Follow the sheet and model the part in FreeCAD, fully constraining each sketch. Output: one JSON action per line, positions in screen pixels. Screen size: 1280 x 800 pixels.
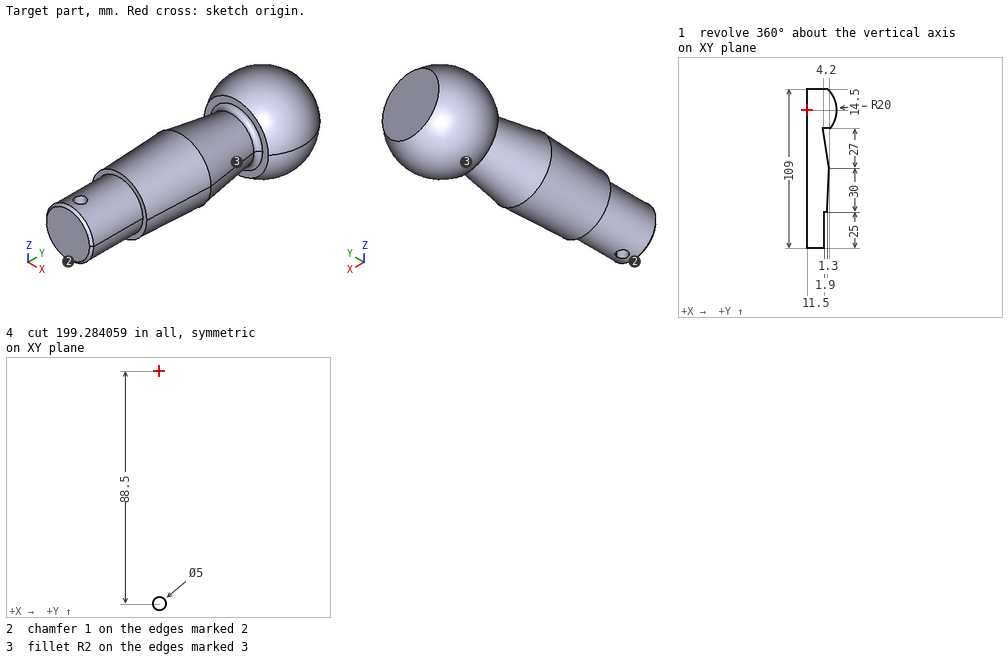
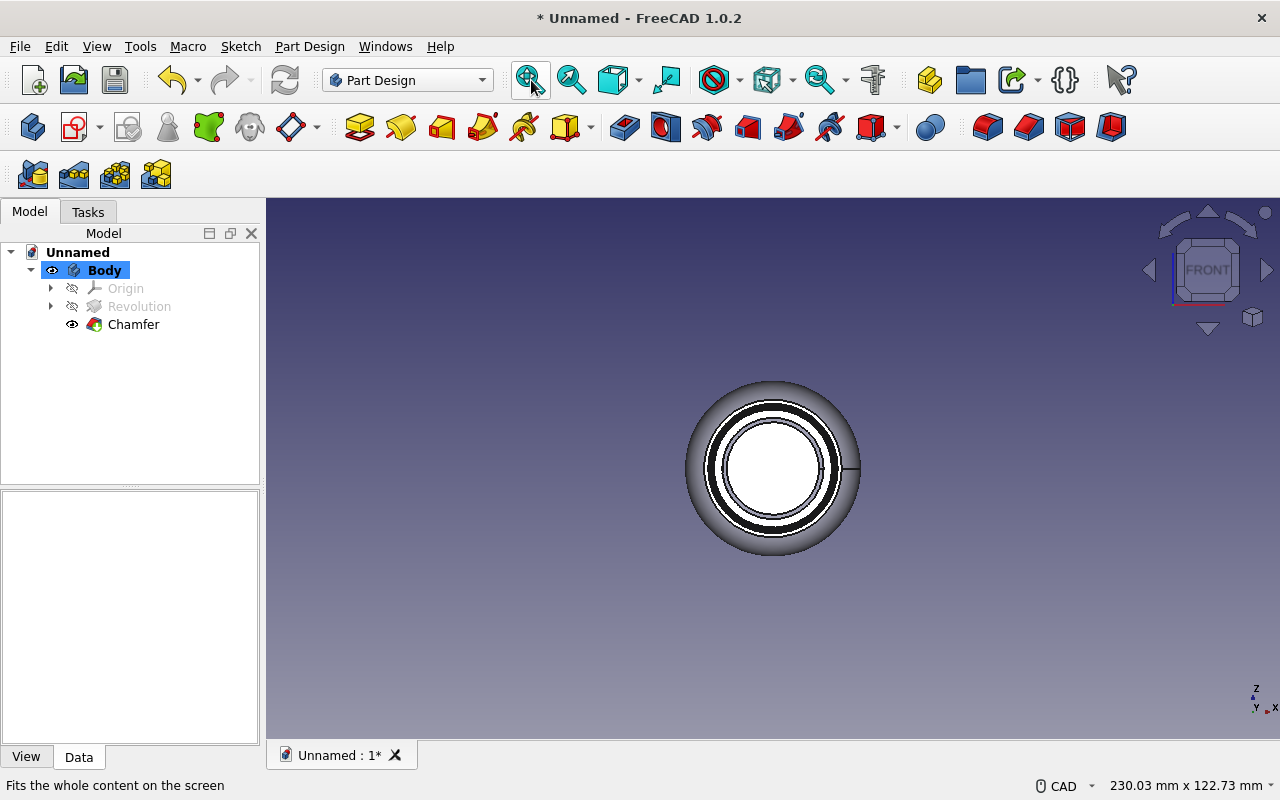
{"action": "key", "text": "3"}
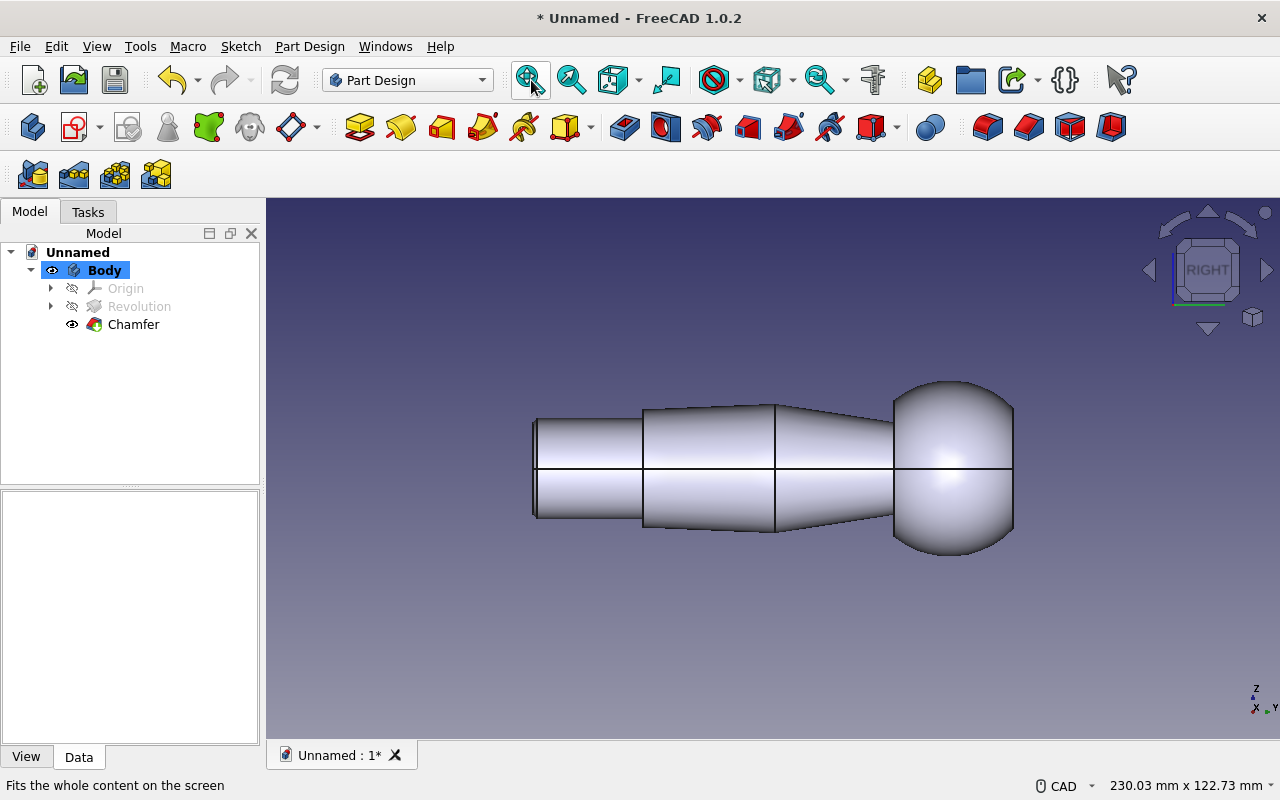
{"action": "key", "text": "5"}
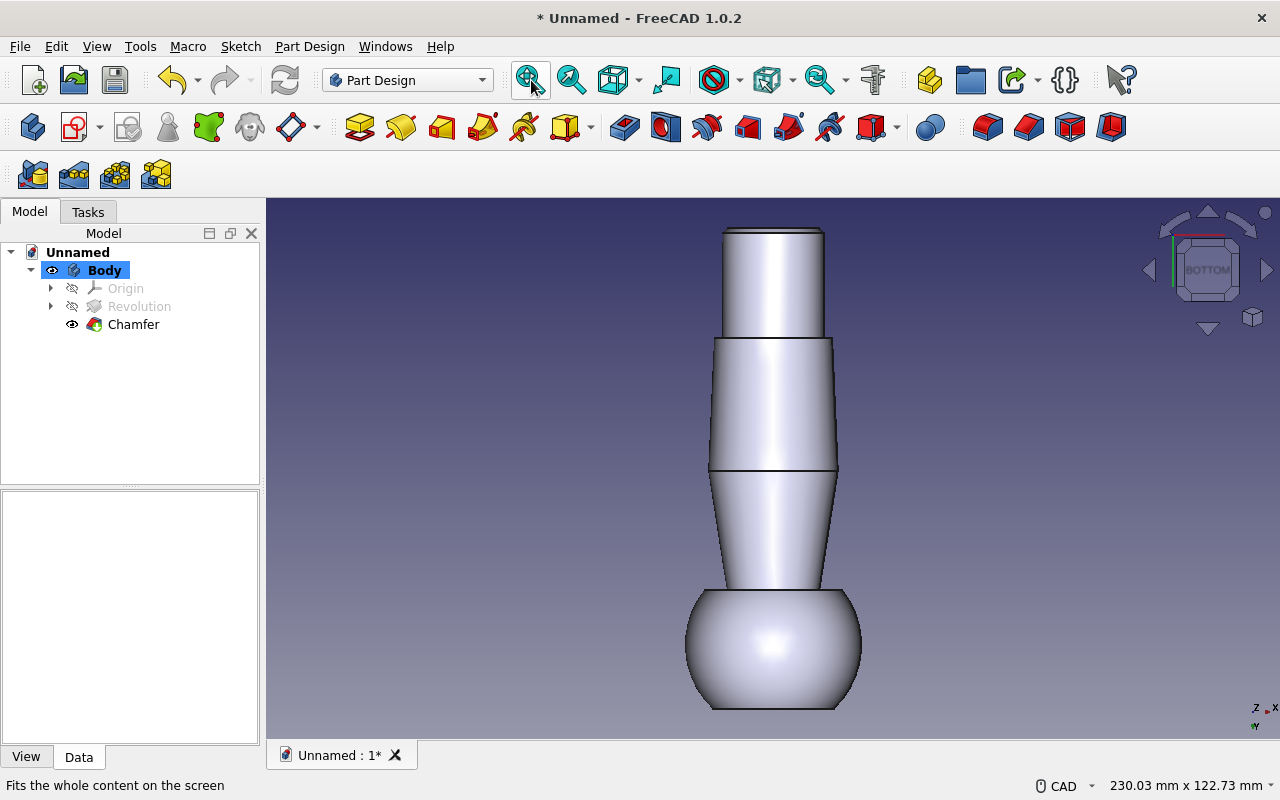
{"action": "key", "text": "4"}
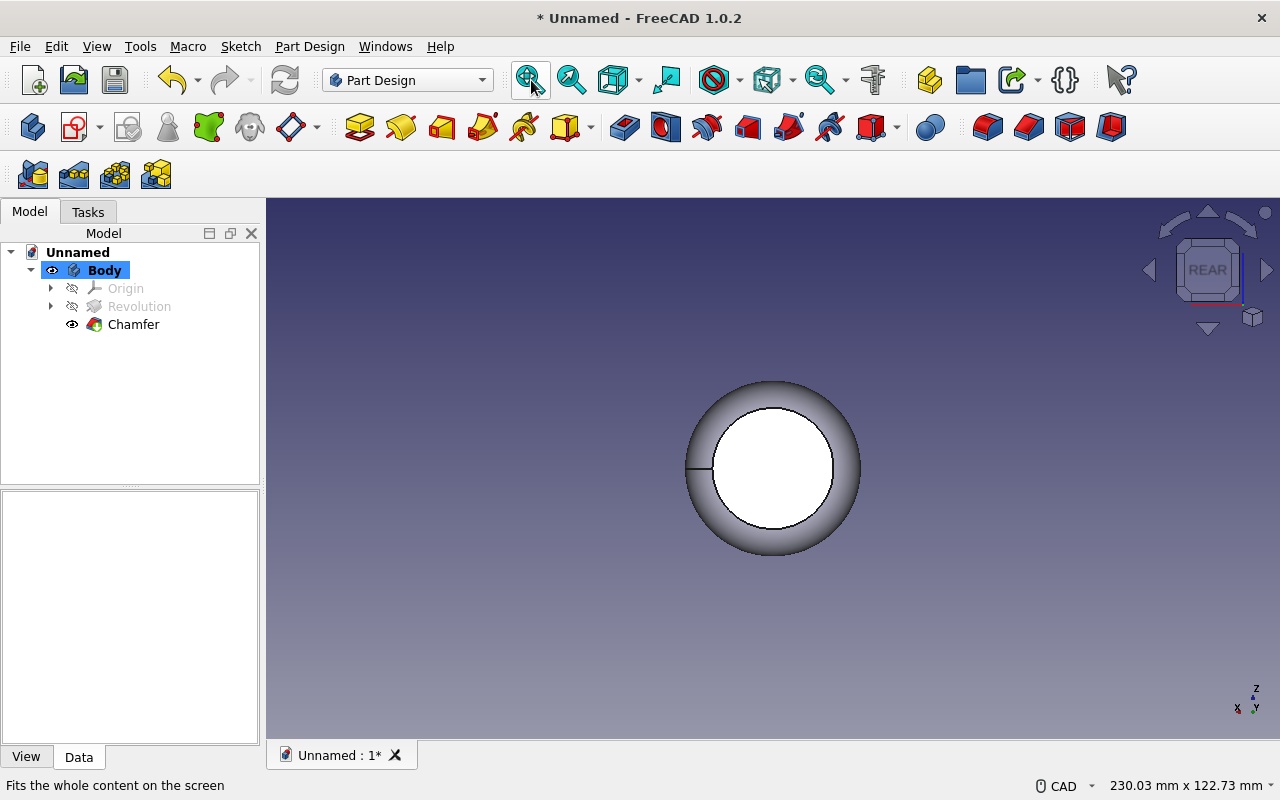
{"action": "left_click", "coordinate": [531, 80]}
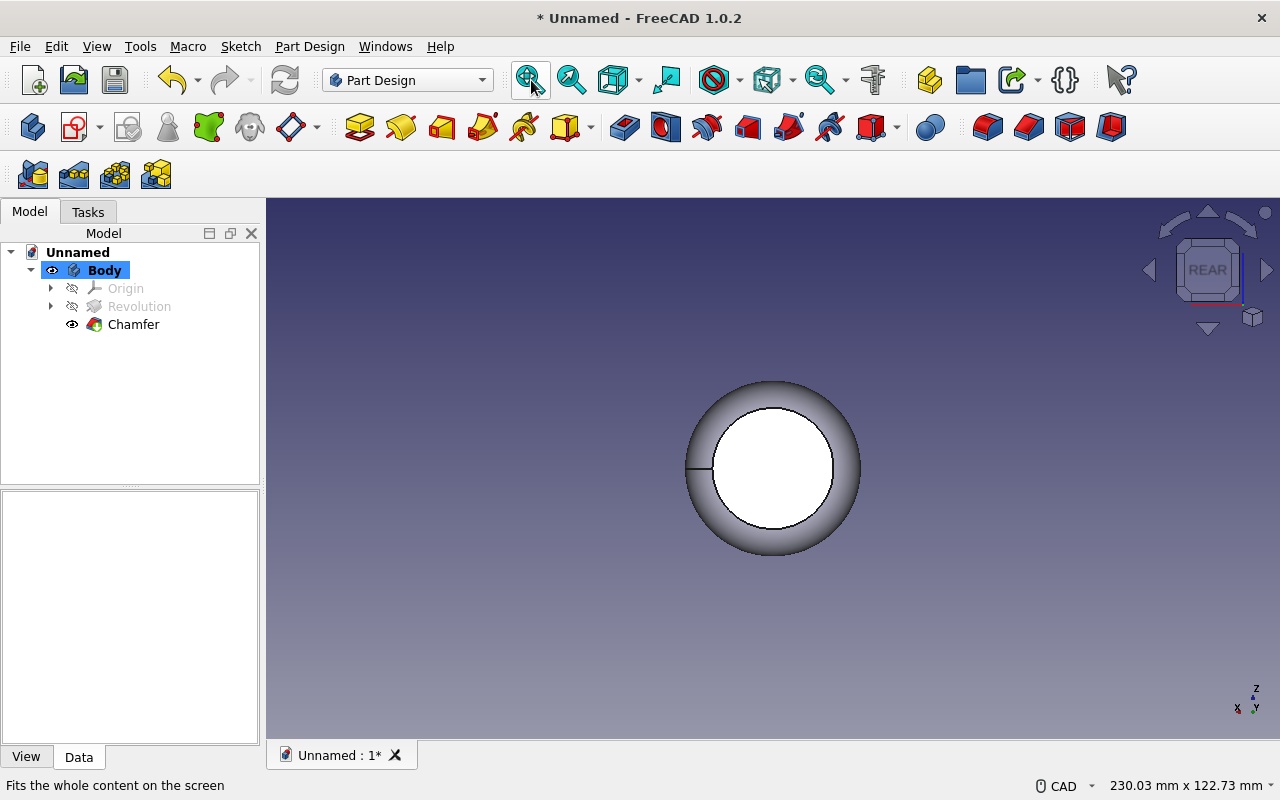
{"action": "key", "text": "6"}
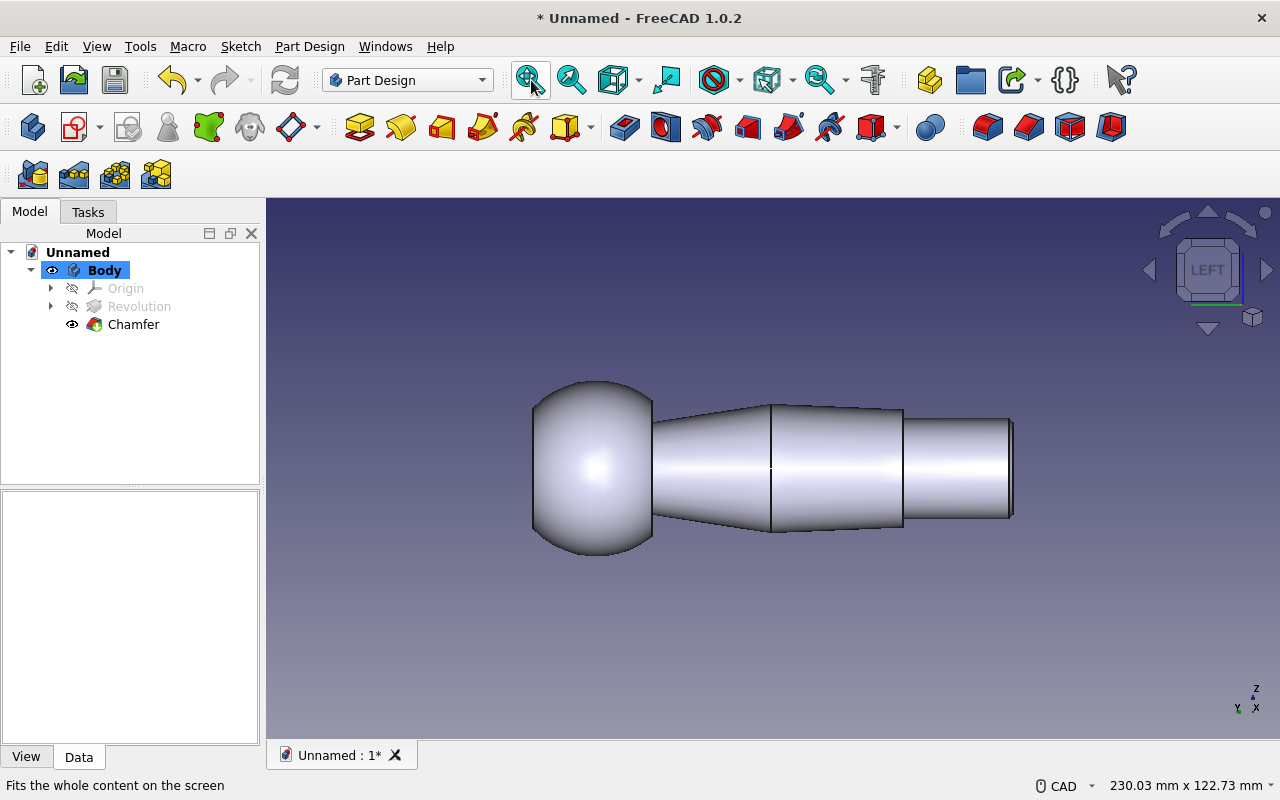
{"action": "key", "text": "v 3"}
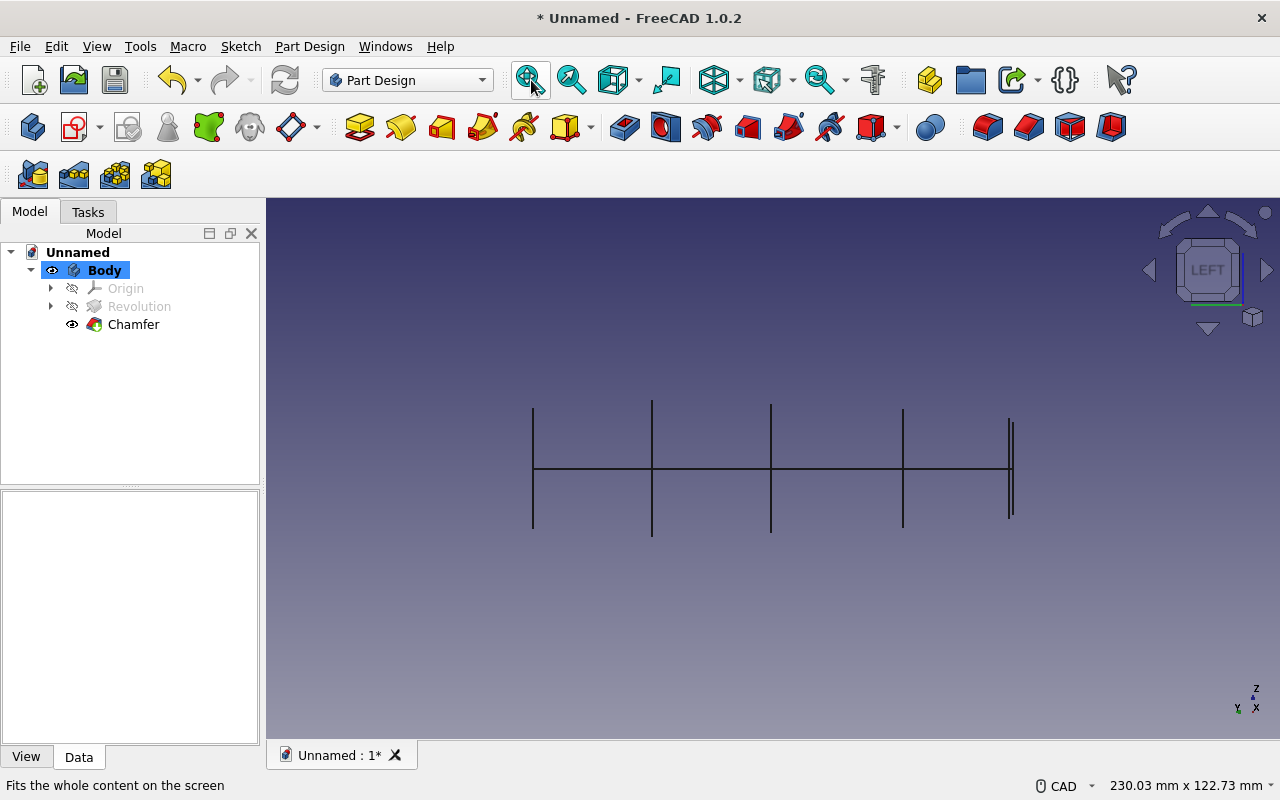
{"action": "key", "text": "0"}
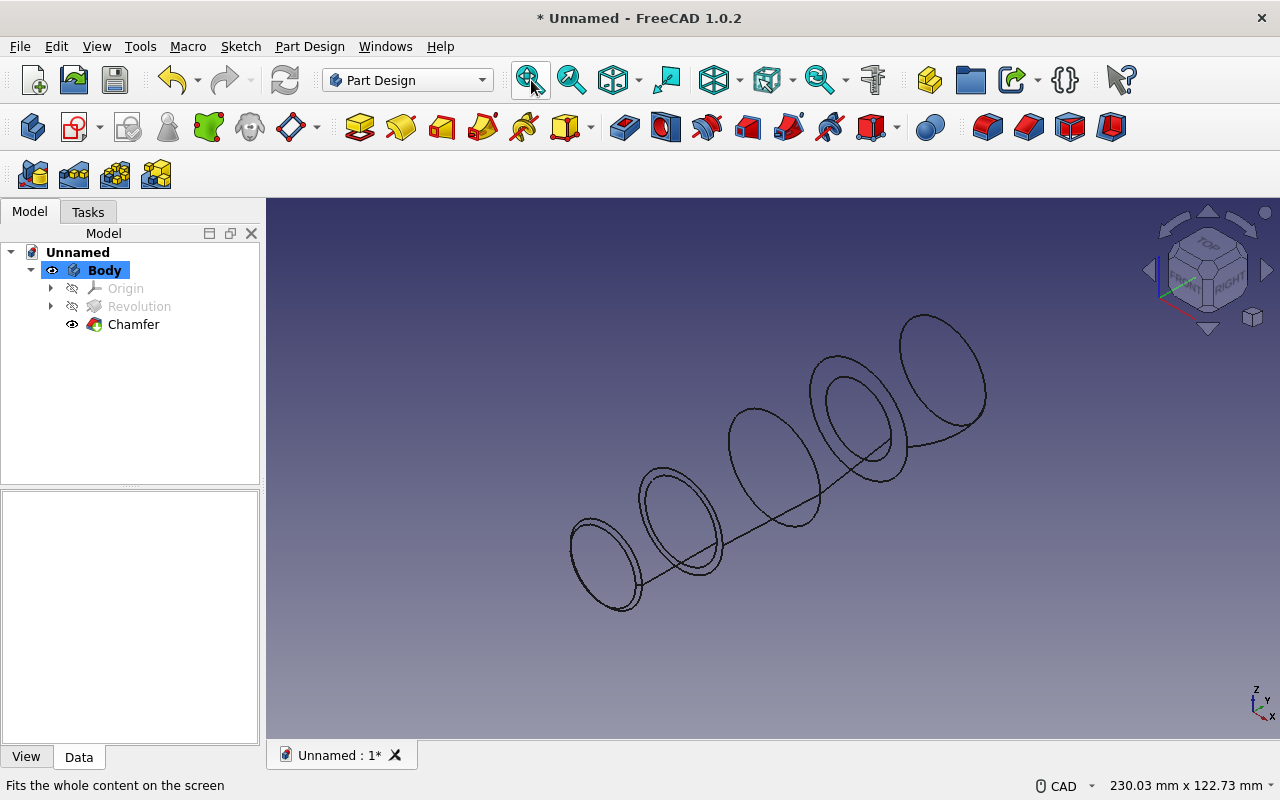
{"action": "left_click", "coordinate": [826, 399]}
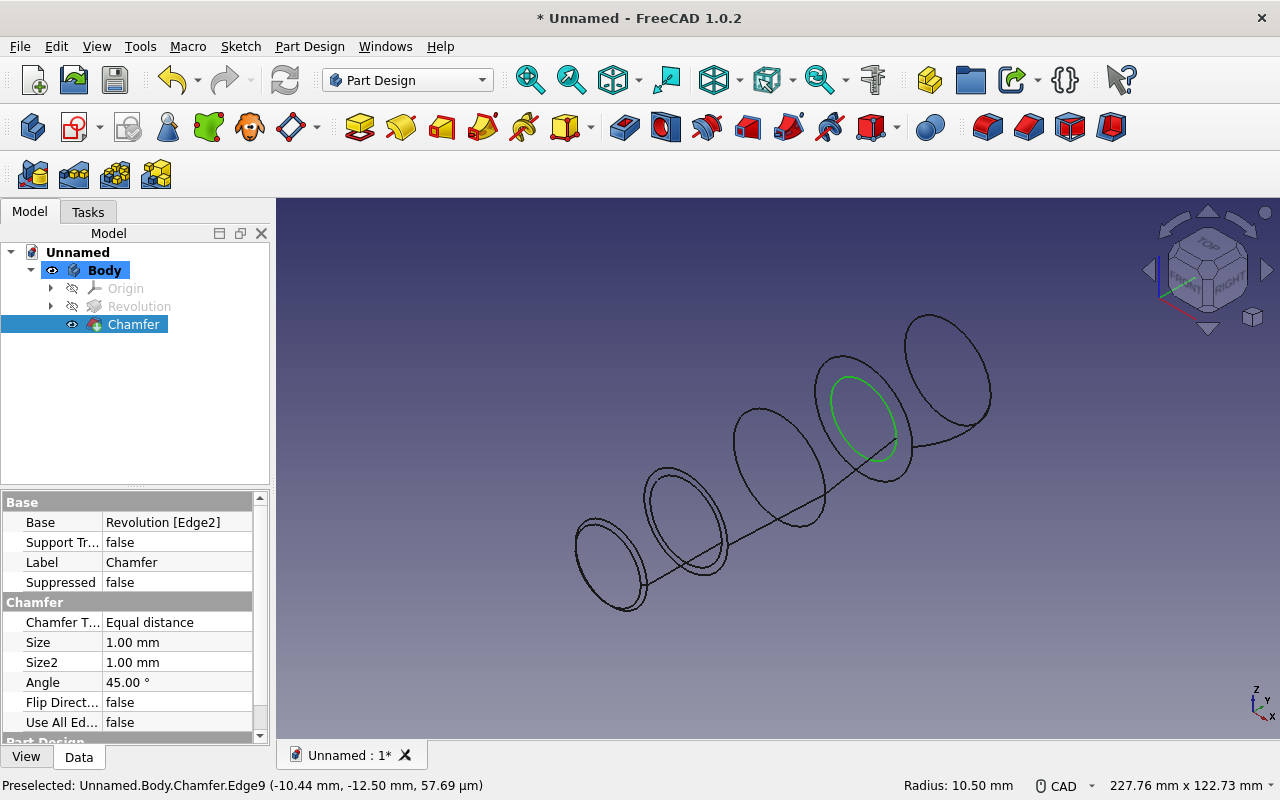
{"action": "key", "text": "v 1"}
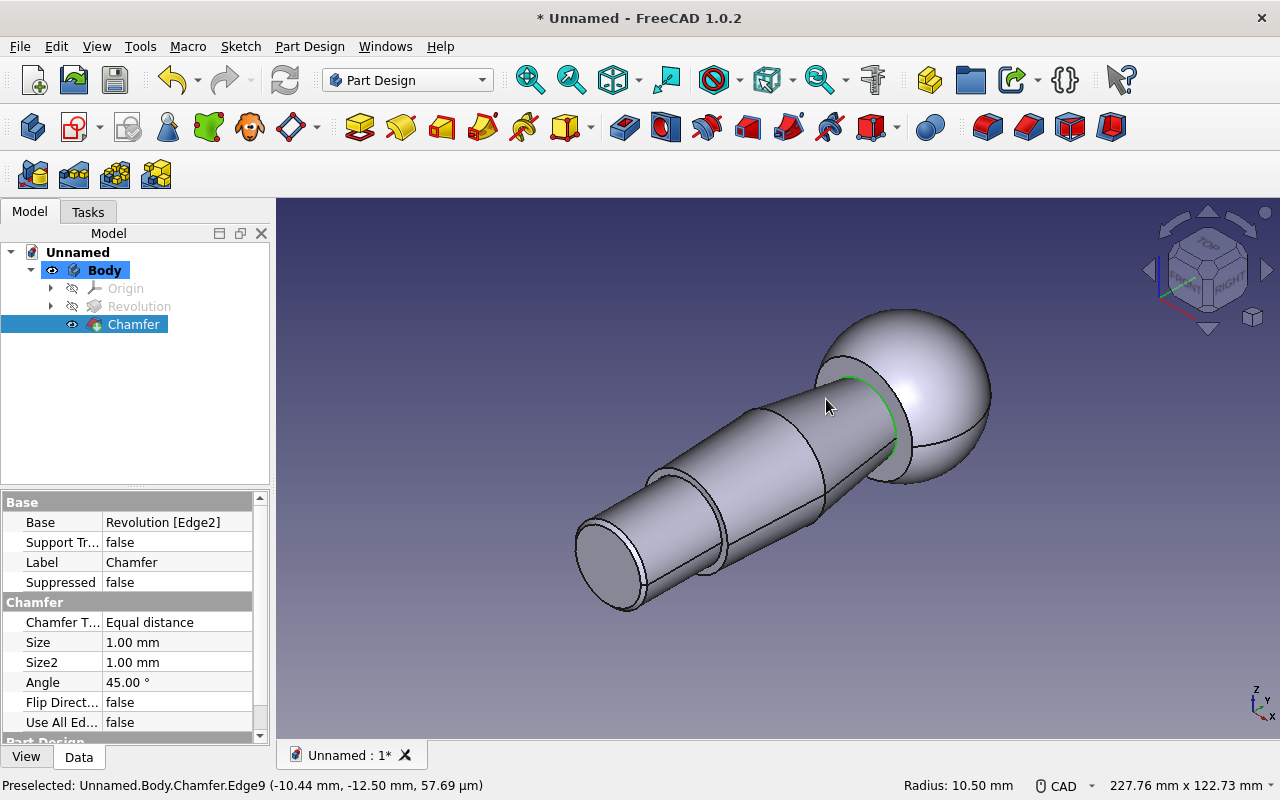
{"action": "left_click", "coordinate": [988, 128]}